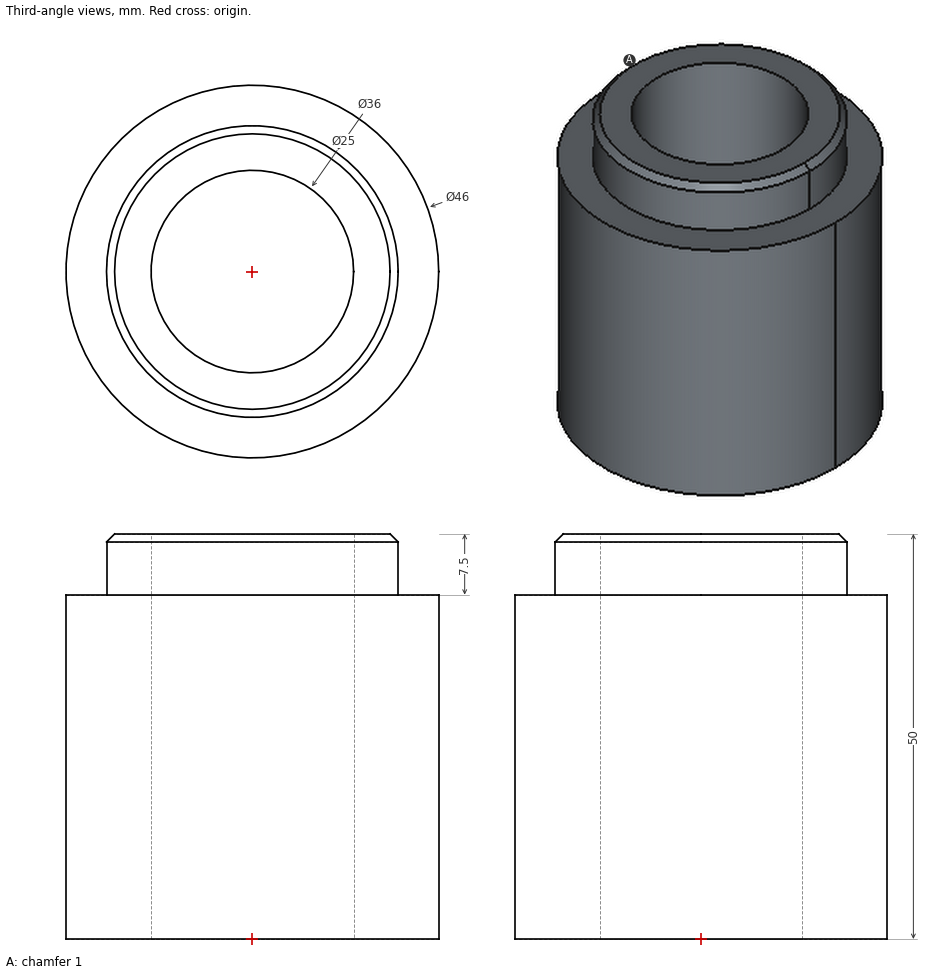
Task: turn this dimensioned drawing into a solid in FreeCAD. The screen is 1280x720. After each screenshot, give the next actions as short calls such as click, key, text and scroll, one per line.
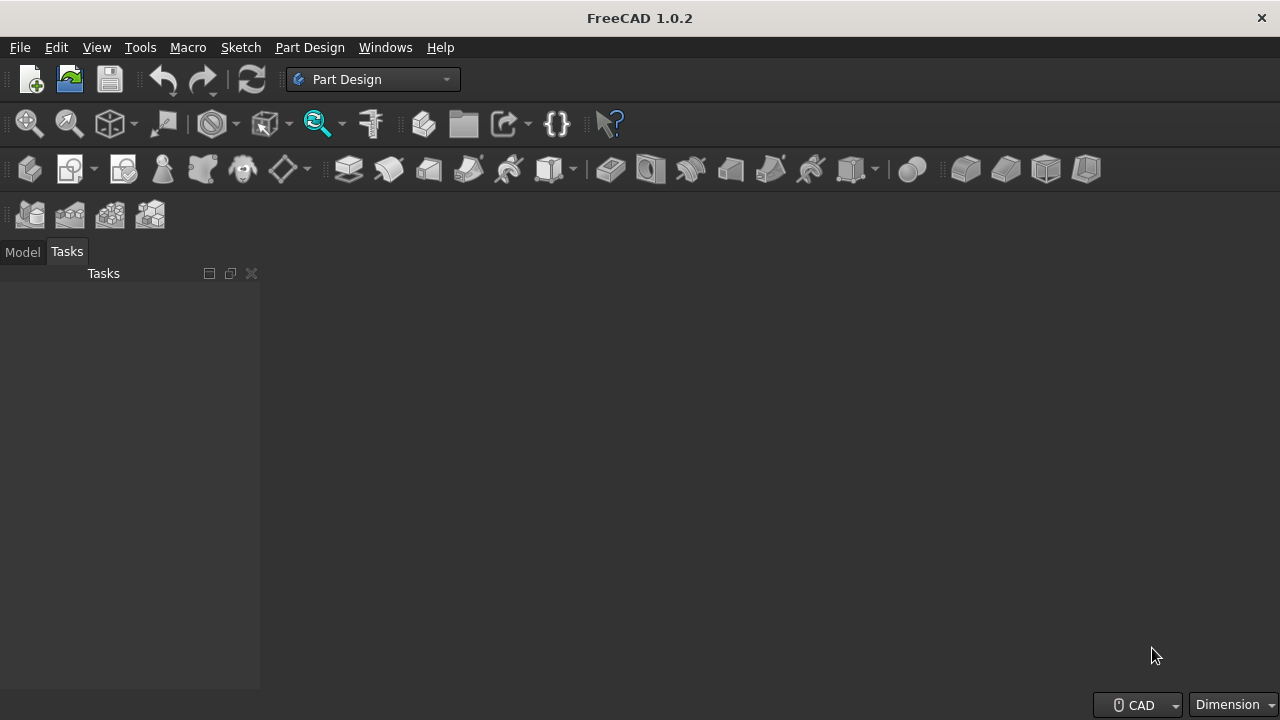
click(30, 80)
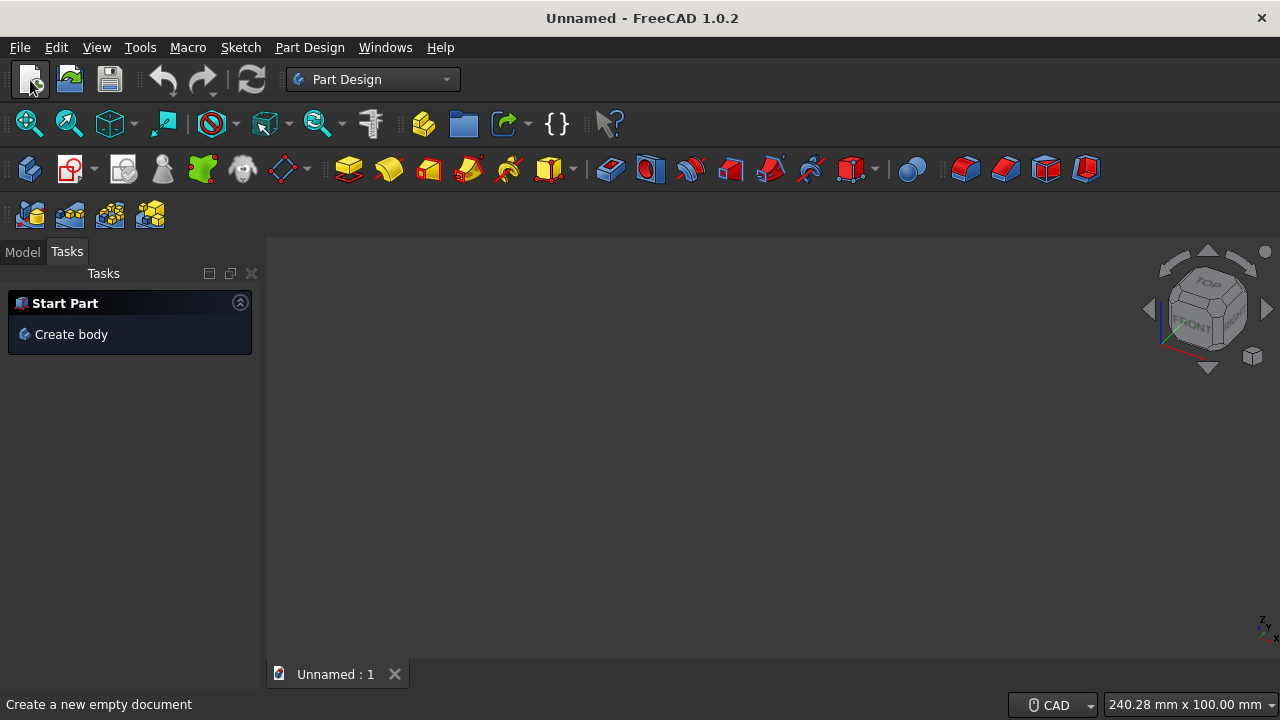
click(70, 170)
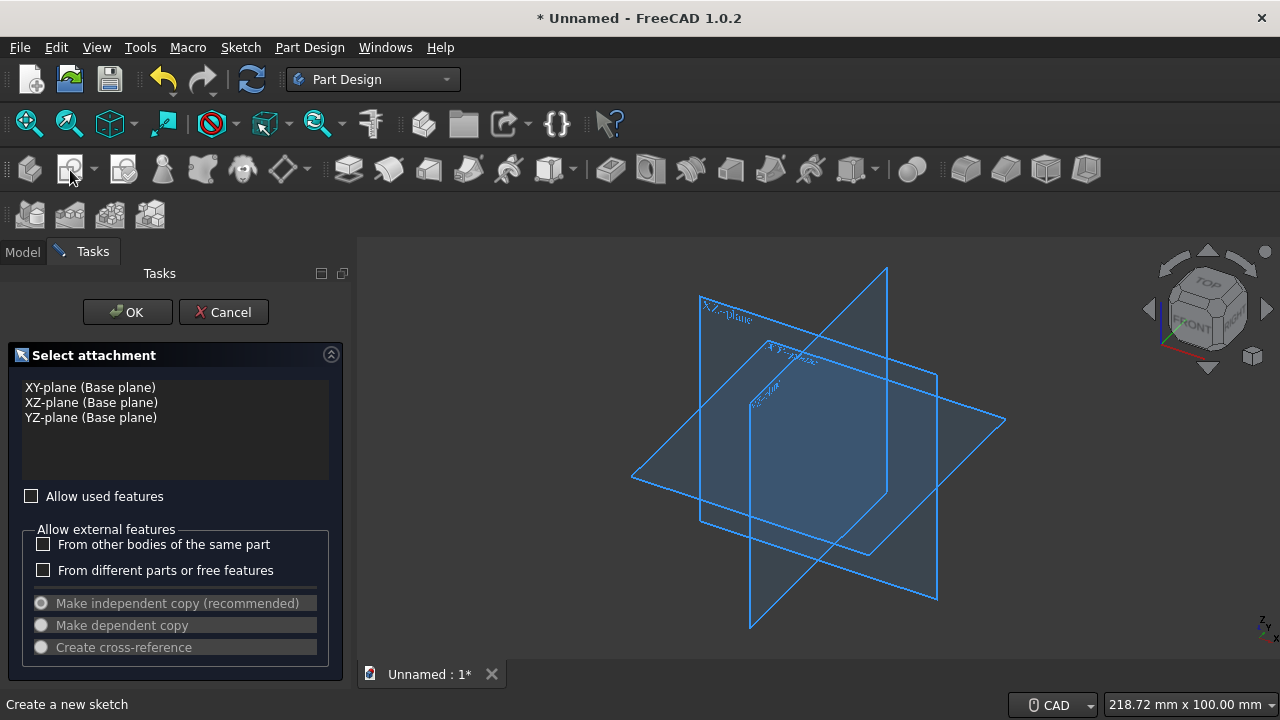
click(82, 388)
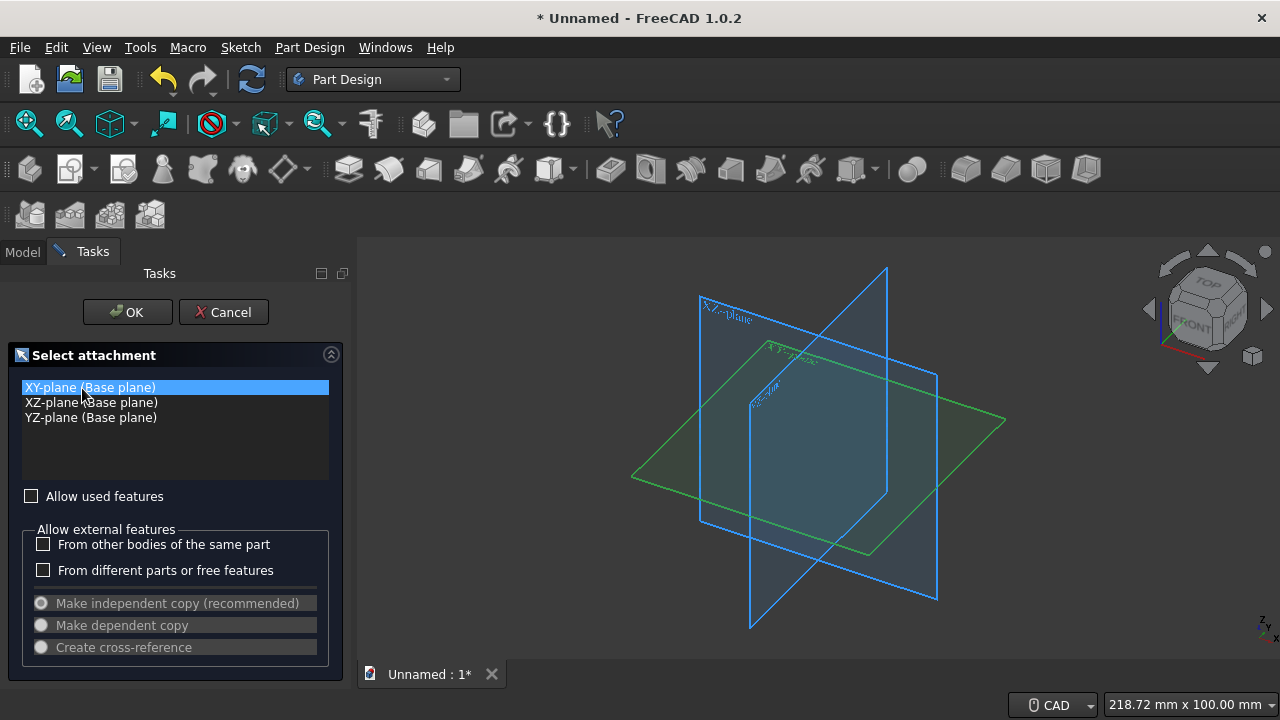
click(128, 312)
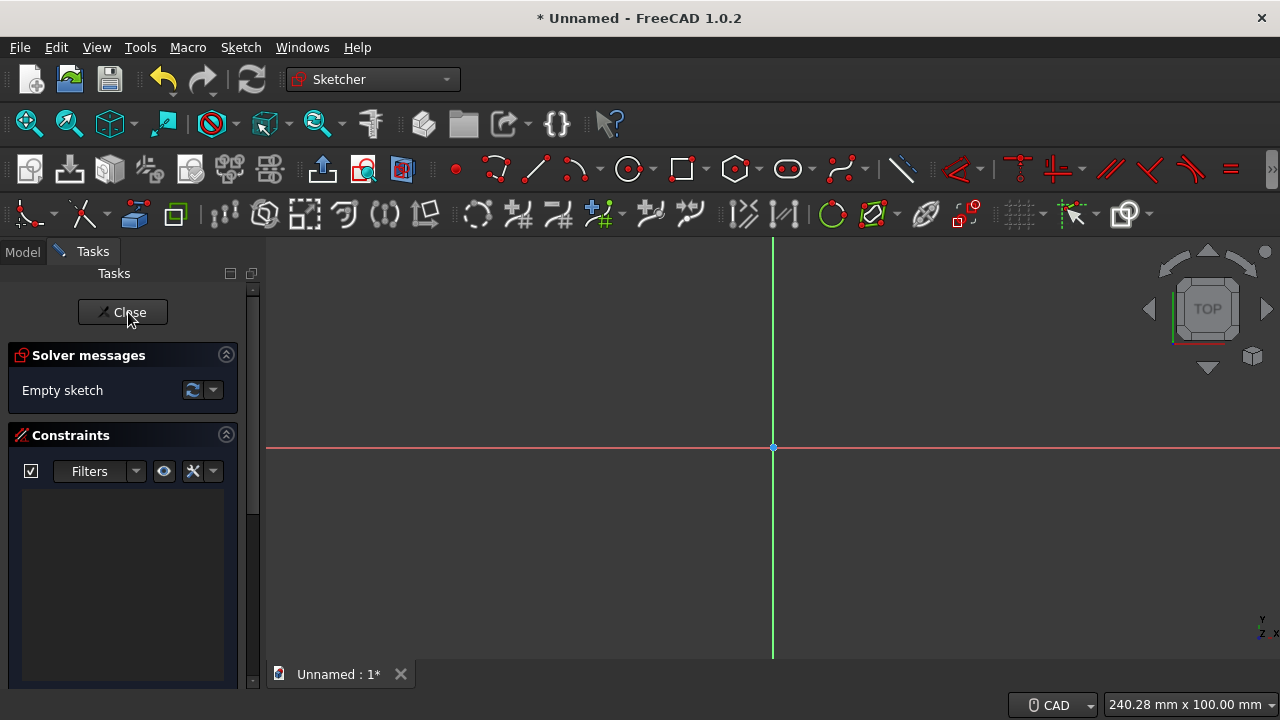
key(g)
key(c)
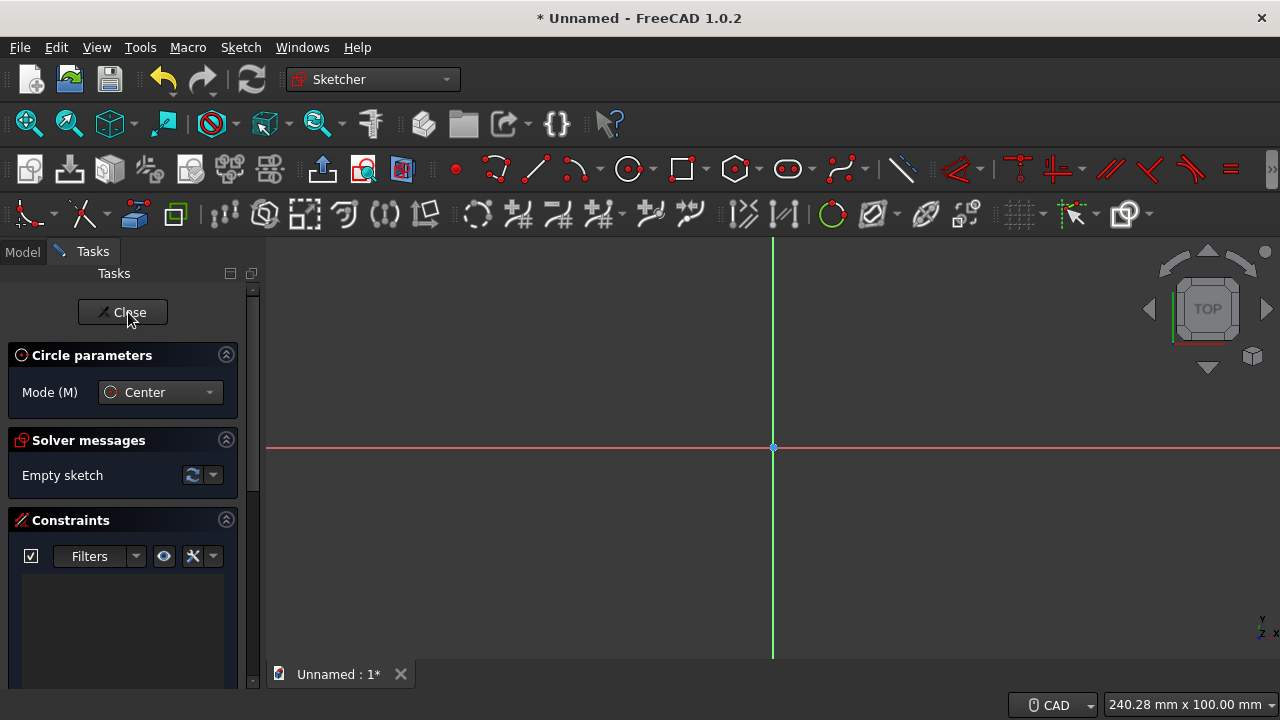
click(773, 448)
move(842, 379)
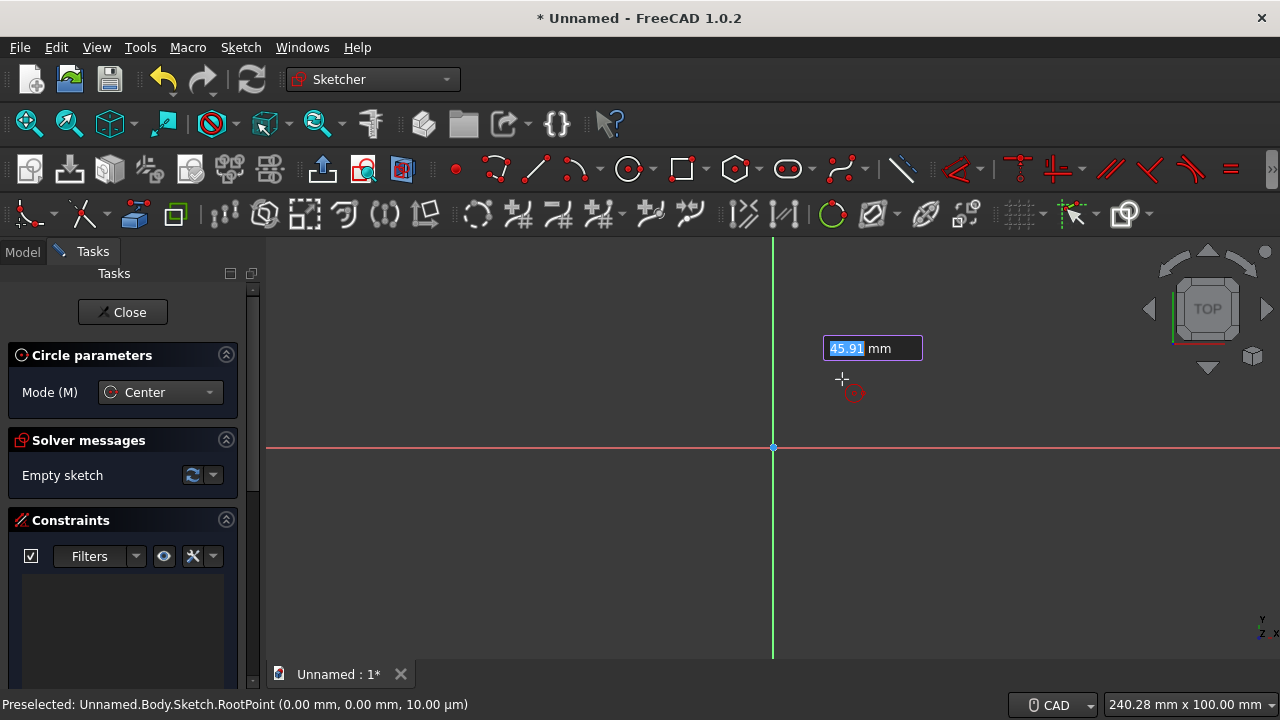
text(46)
key(Return)
key(Escape)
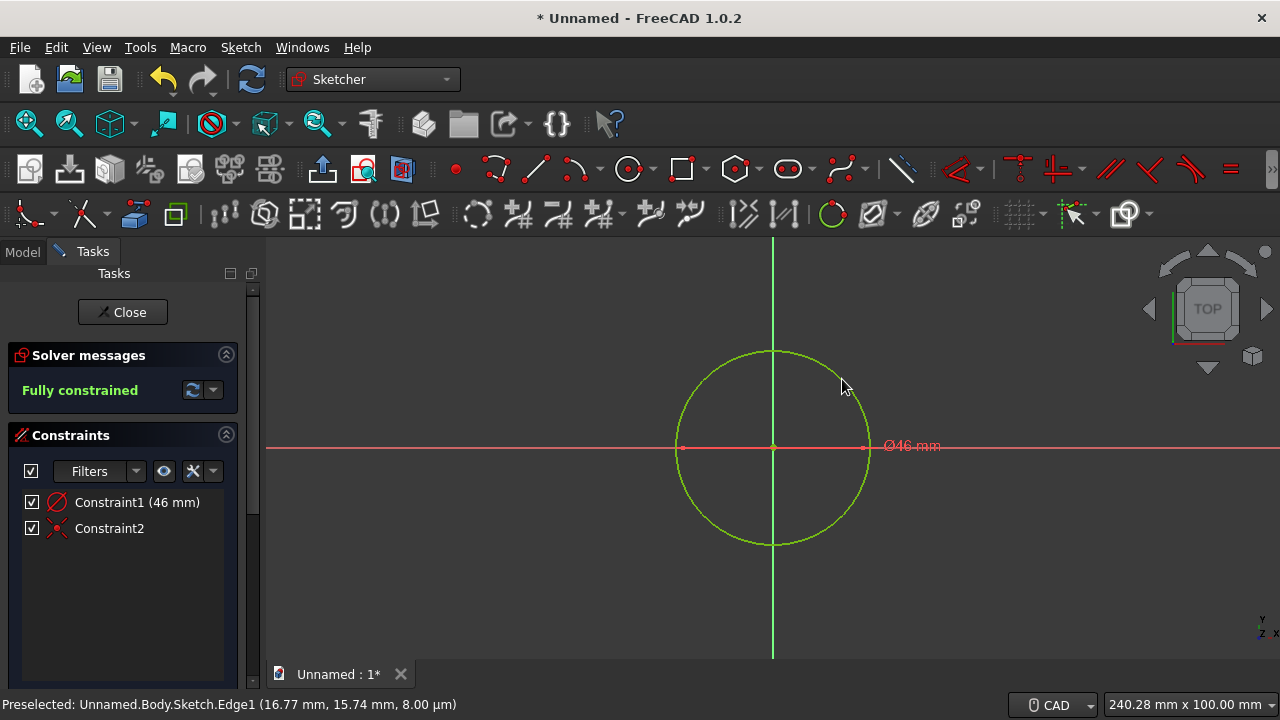
click(123, 312)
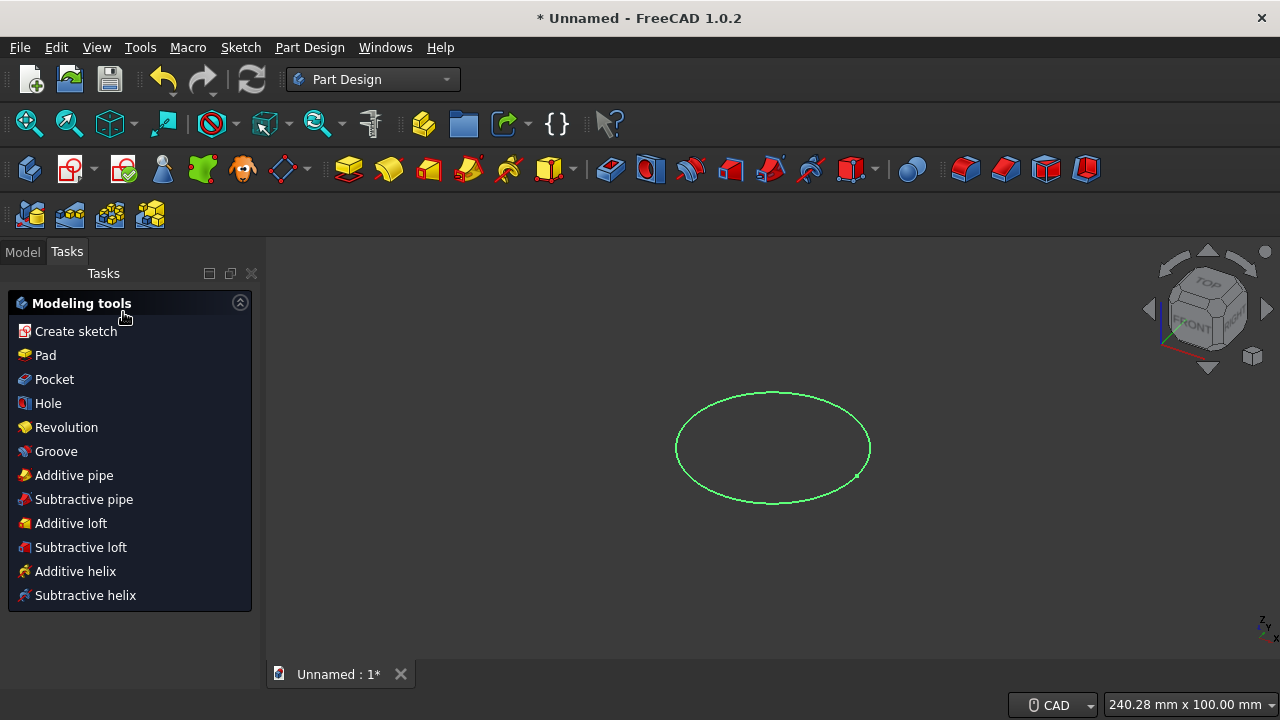
click(350, 170)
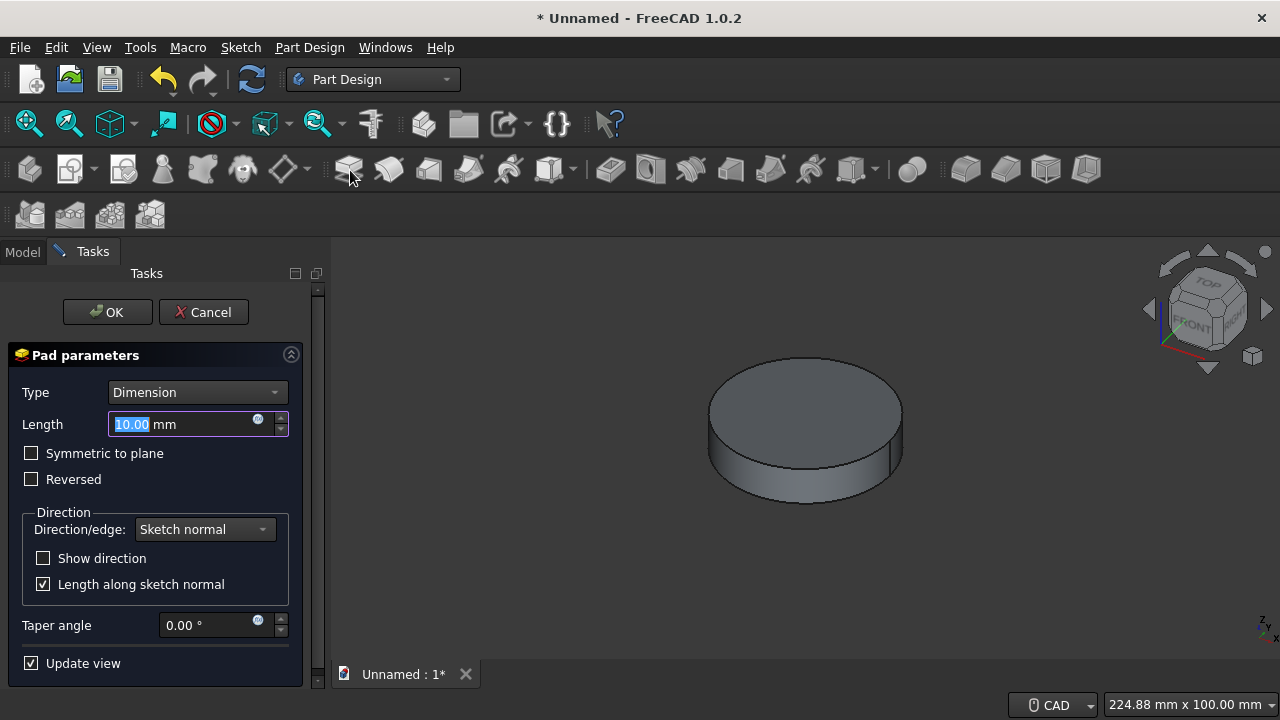
text(50)
key(Tab)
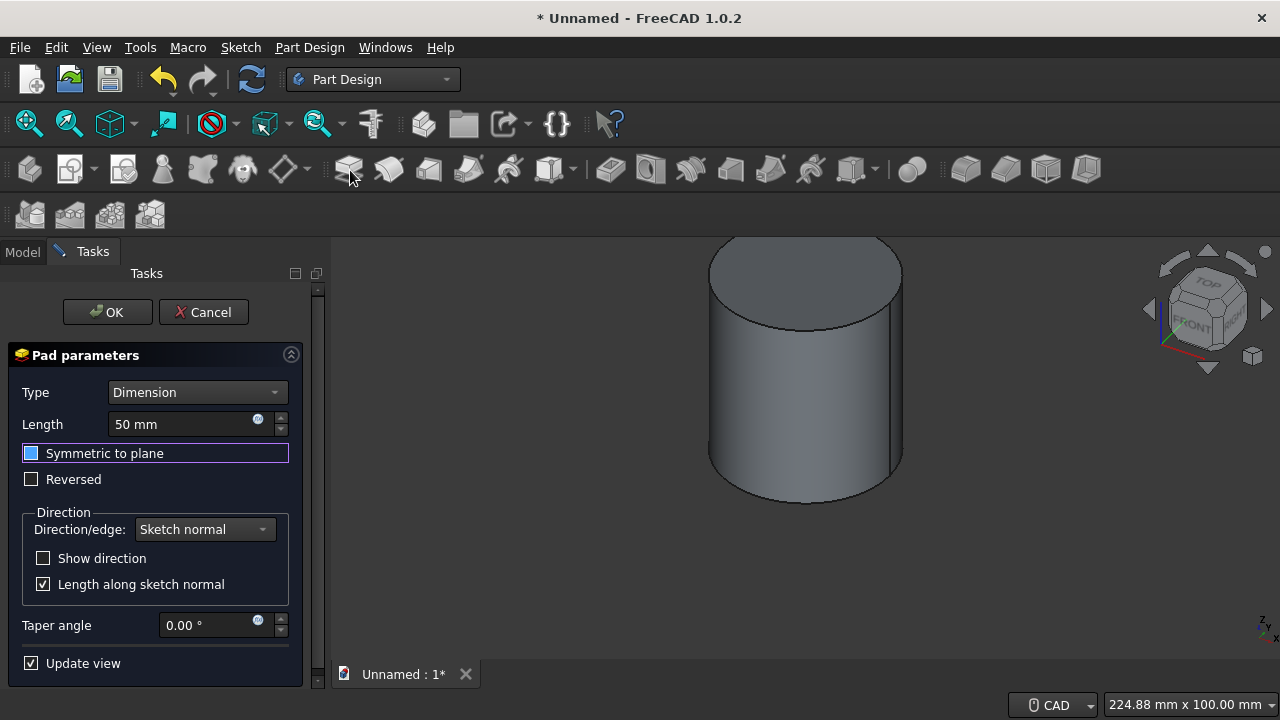
click(108, 312)